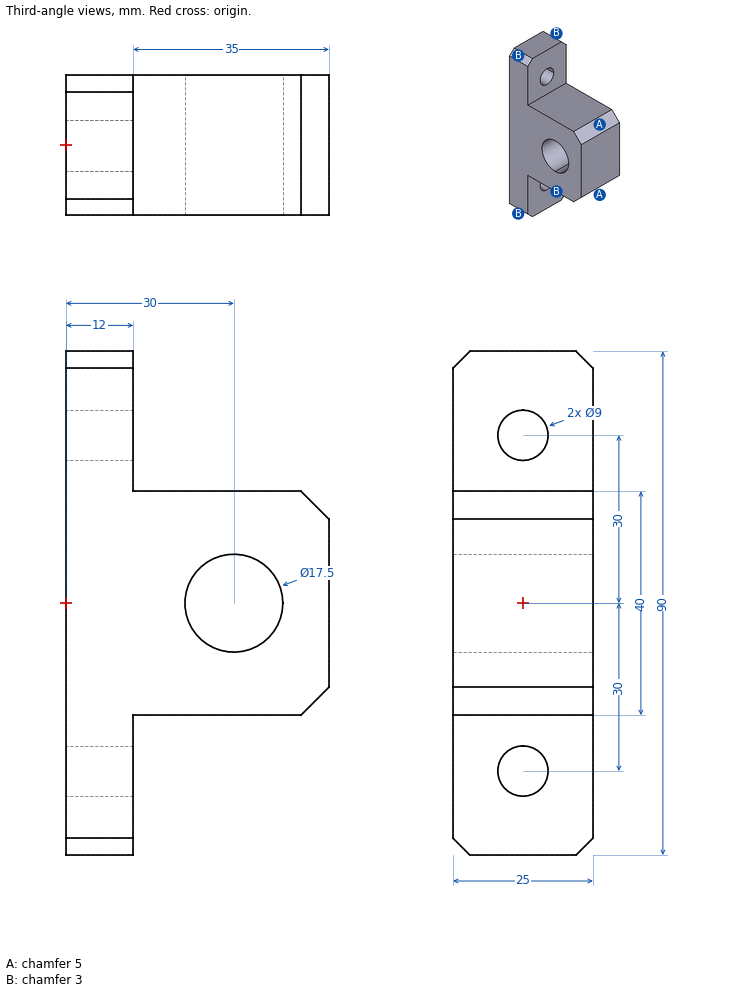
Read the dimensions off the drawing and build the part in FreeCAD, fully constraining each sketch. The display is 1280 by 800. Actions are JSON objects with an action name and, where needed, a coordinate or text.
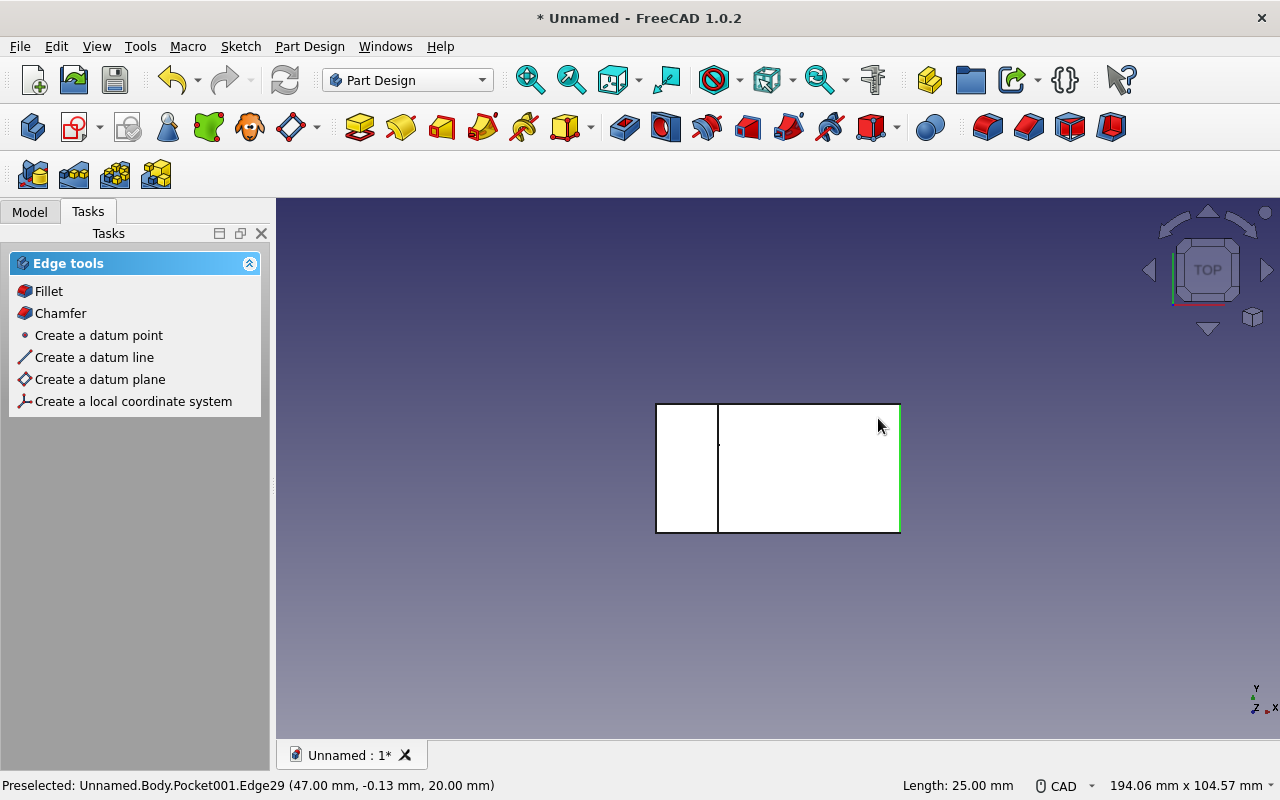
{"action": "left_click", "coordinate": [531, 80]}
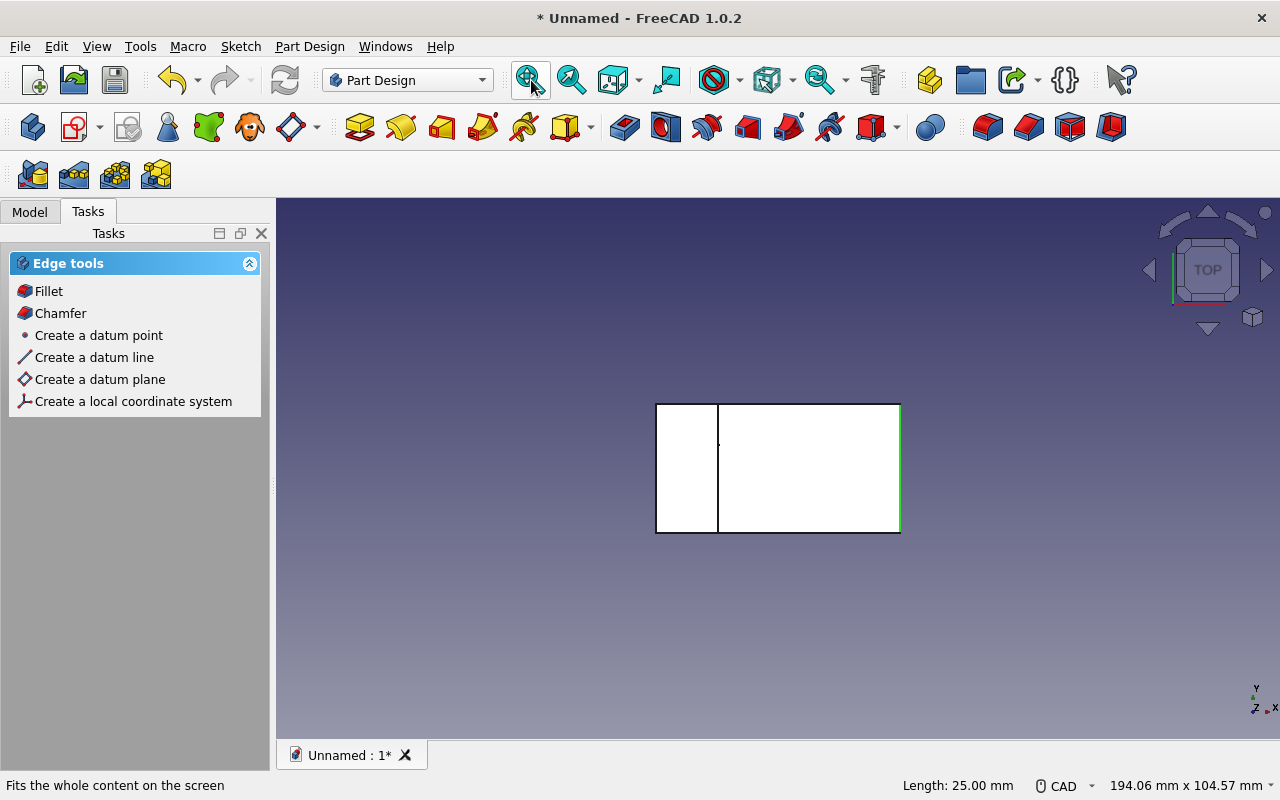
{"action": "key", "text": "1"}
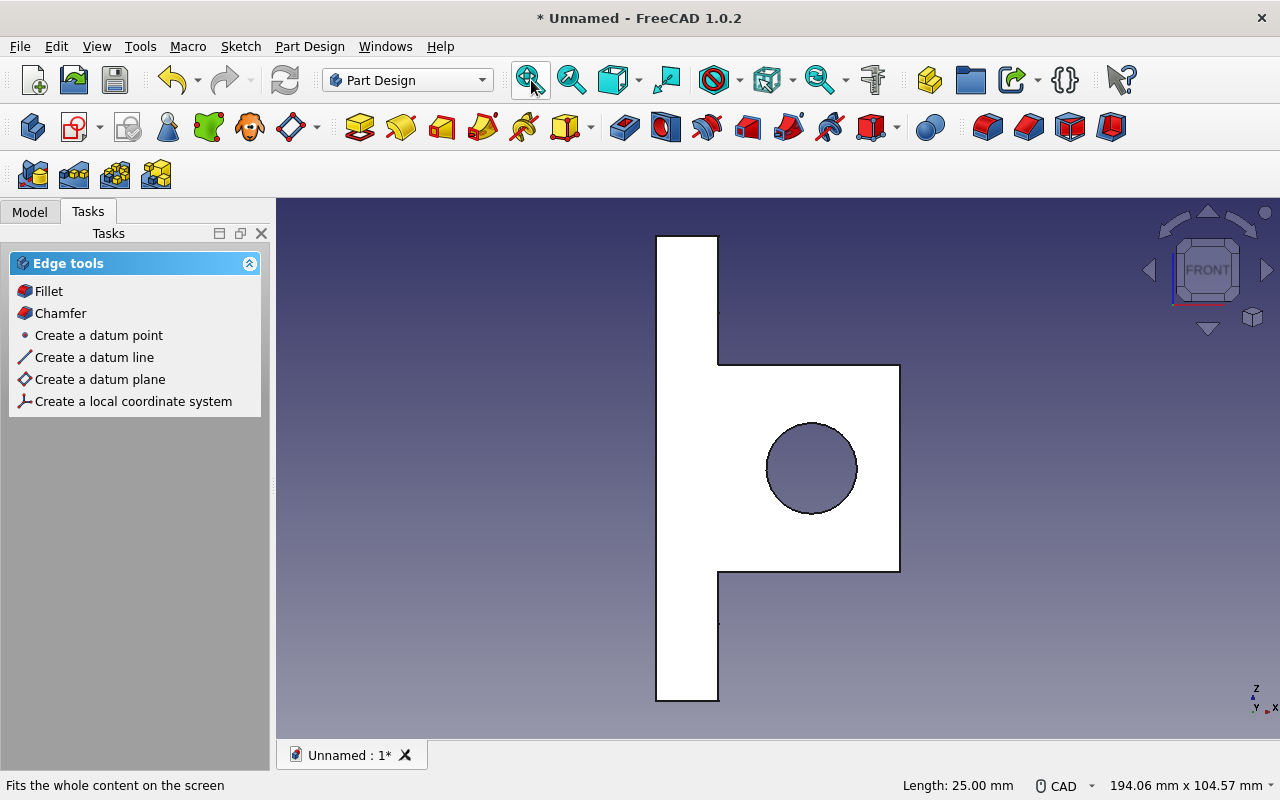
{"action": "key", "text": "3"}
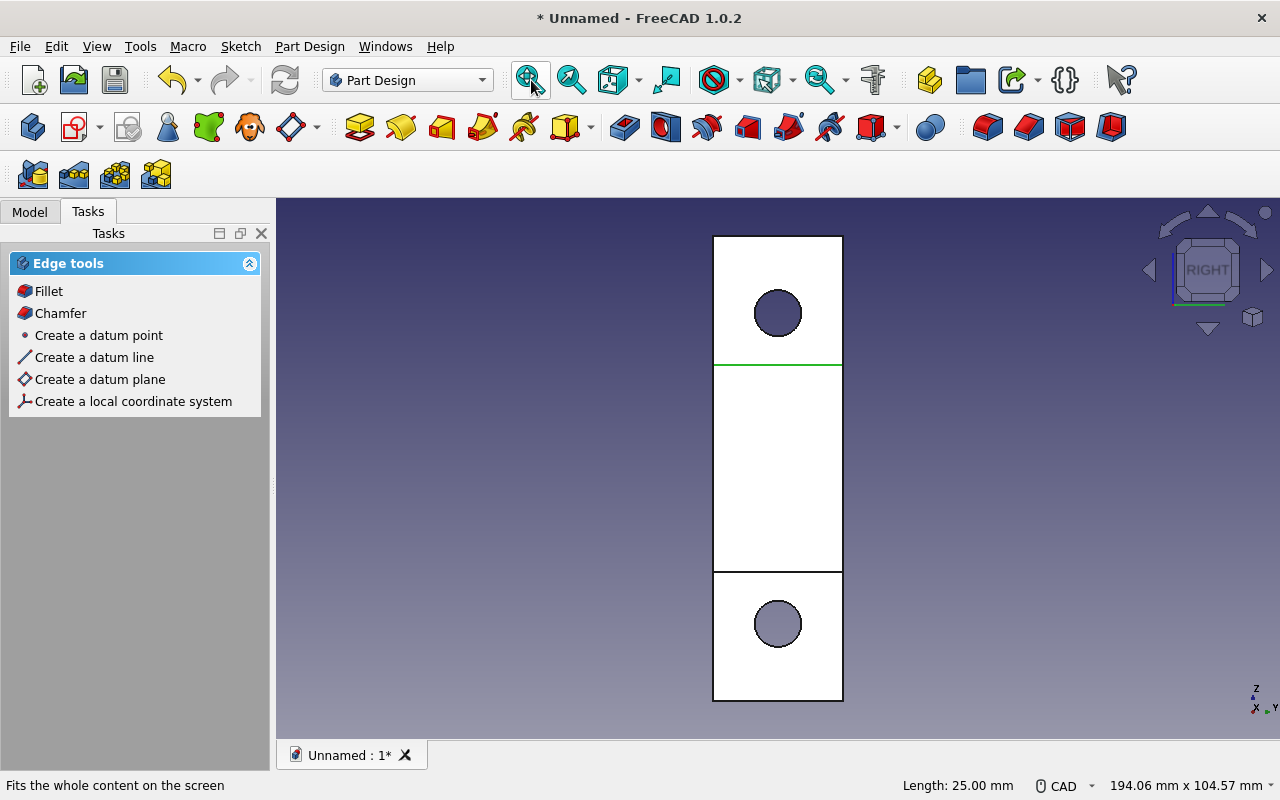
{"action": "left_click", "coordinate": [778, 571], "text": "ctrl"}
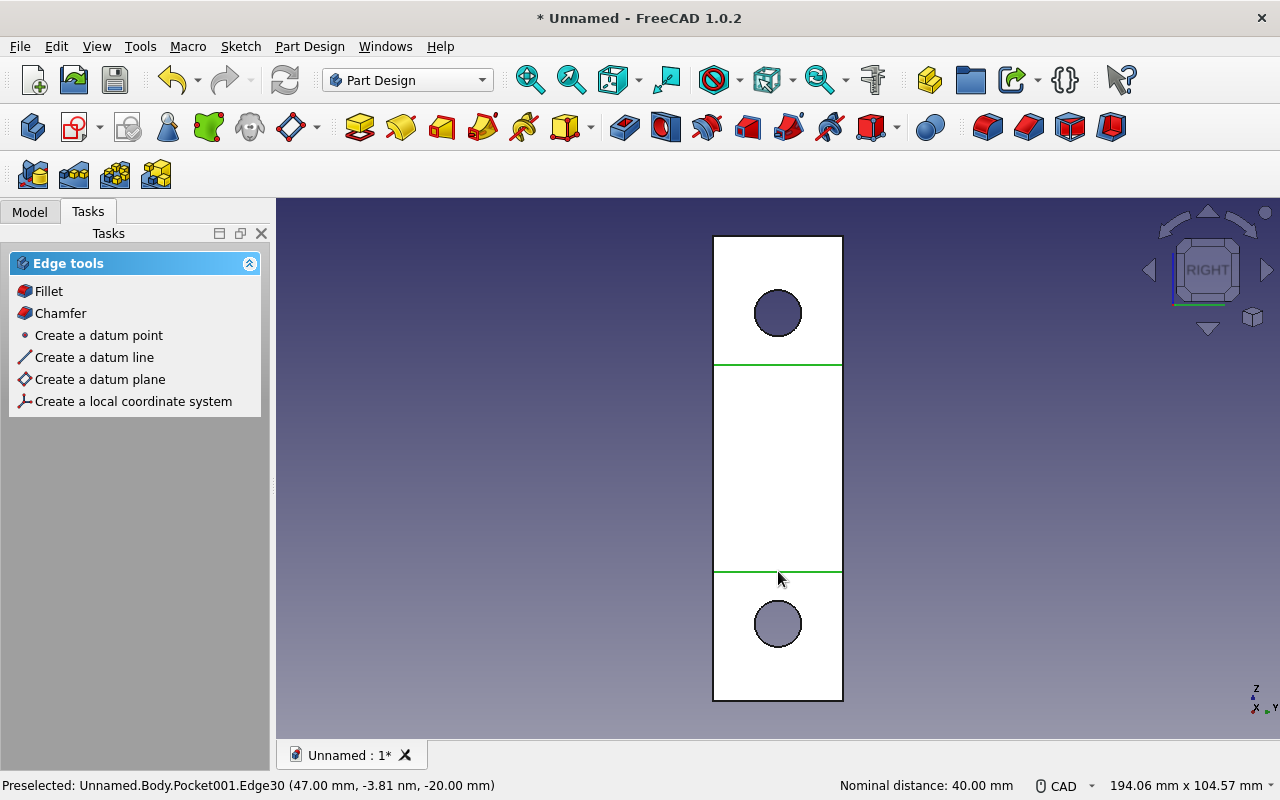
{"action": "left_click", "coordinate": [1029, 128]}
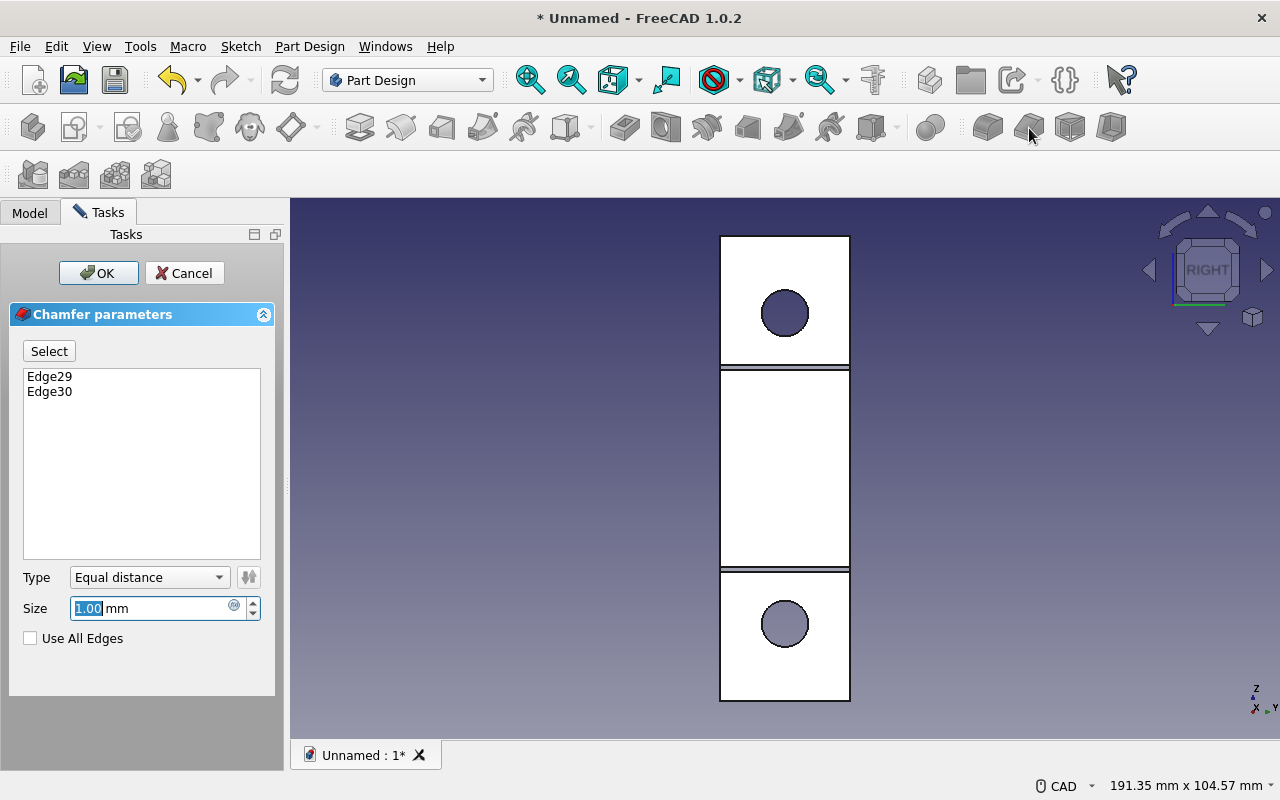
{"action": "type", "text": "5"}
{"action": "key", "text": "Tab"}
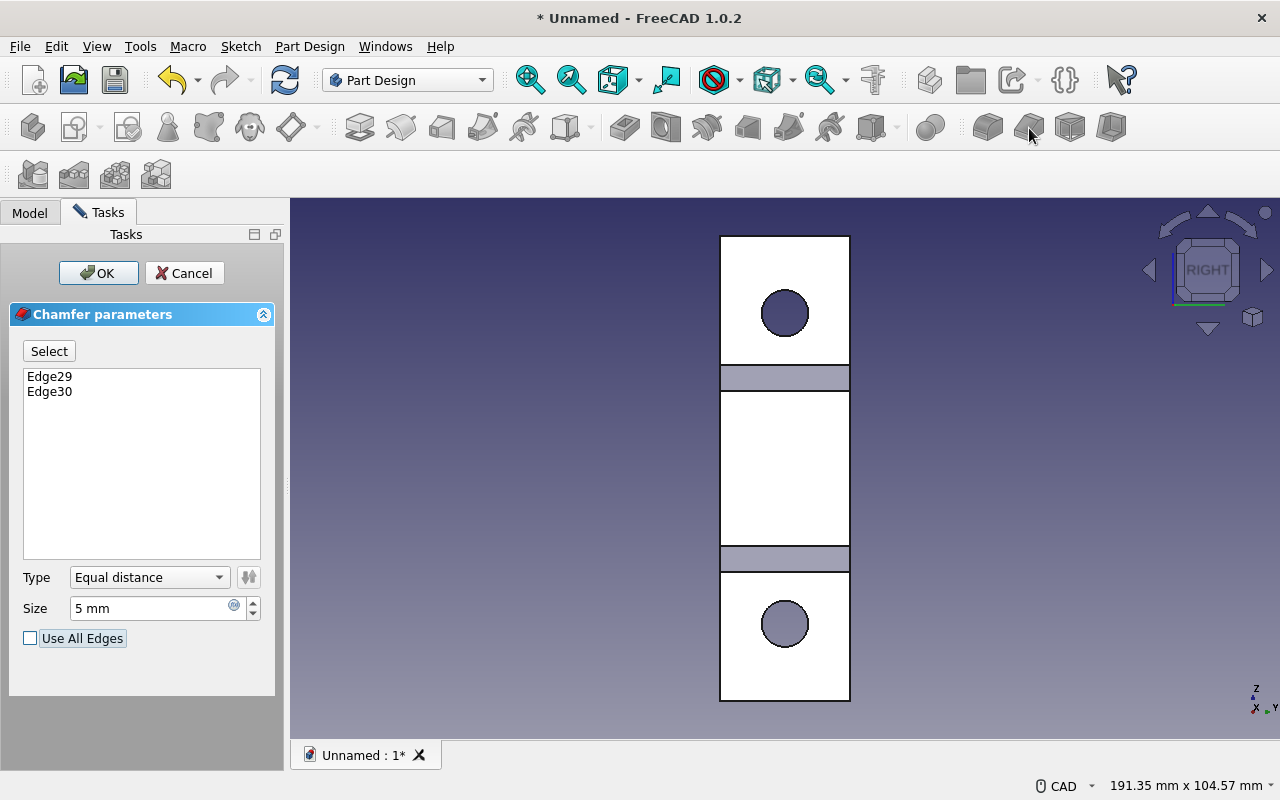
{"action": "left_click", "coordinate": [99, 273]}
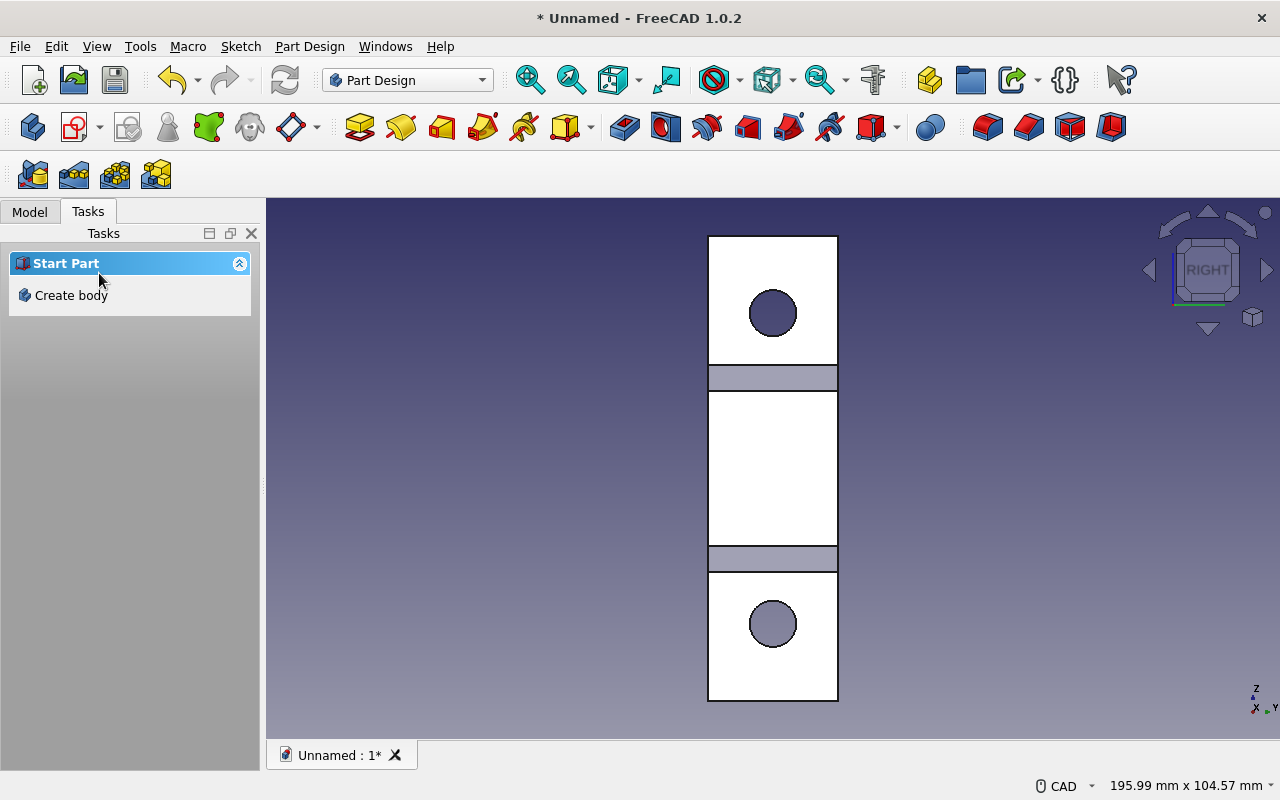
{"action": "key", "text": "0"}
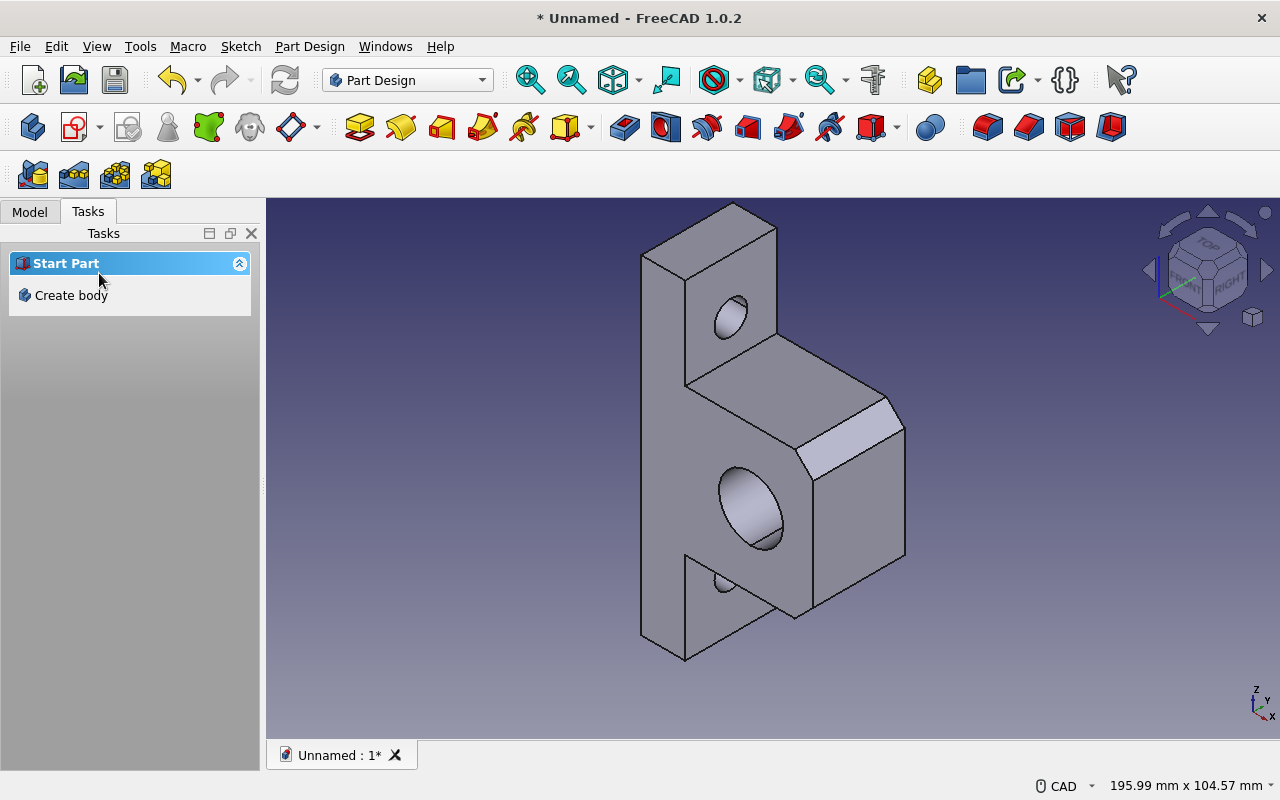
{"action": "left_click", "coordinate": [663, 267]}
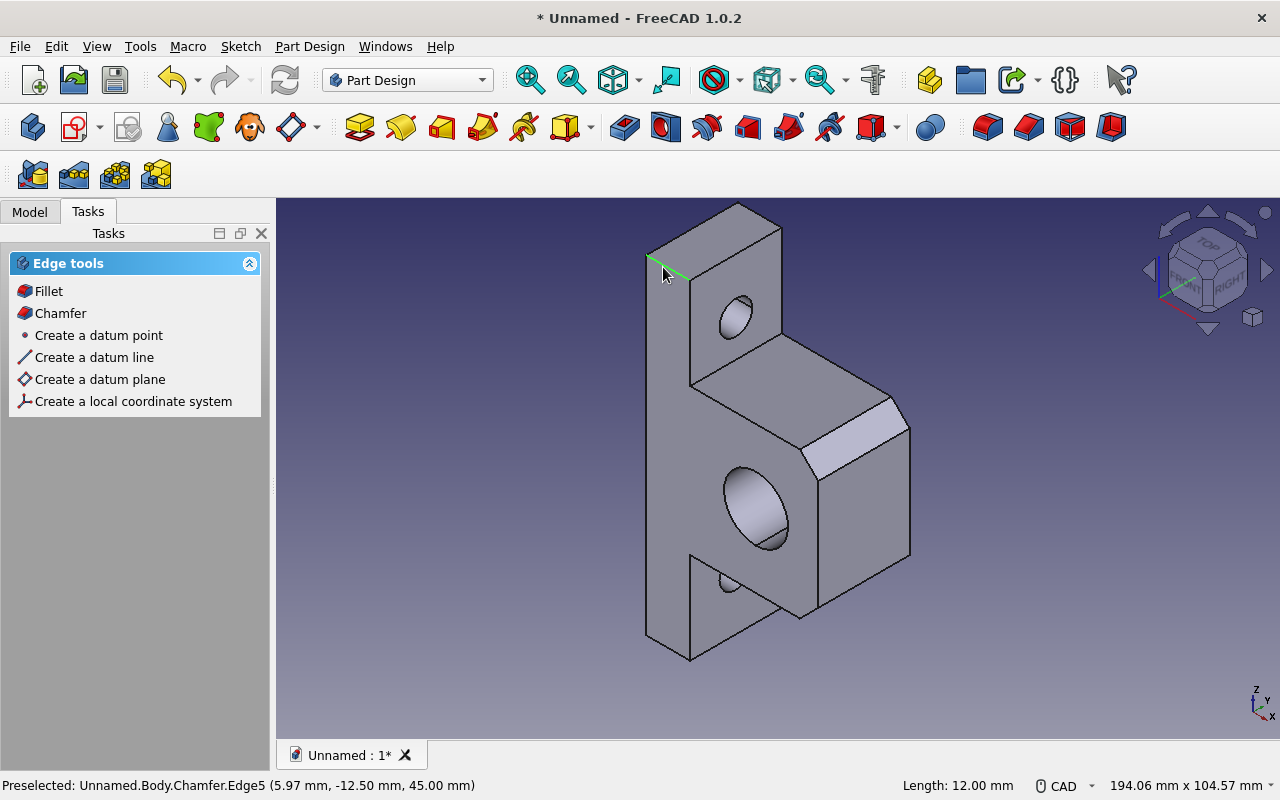
{"action": "key", "text": "2"}